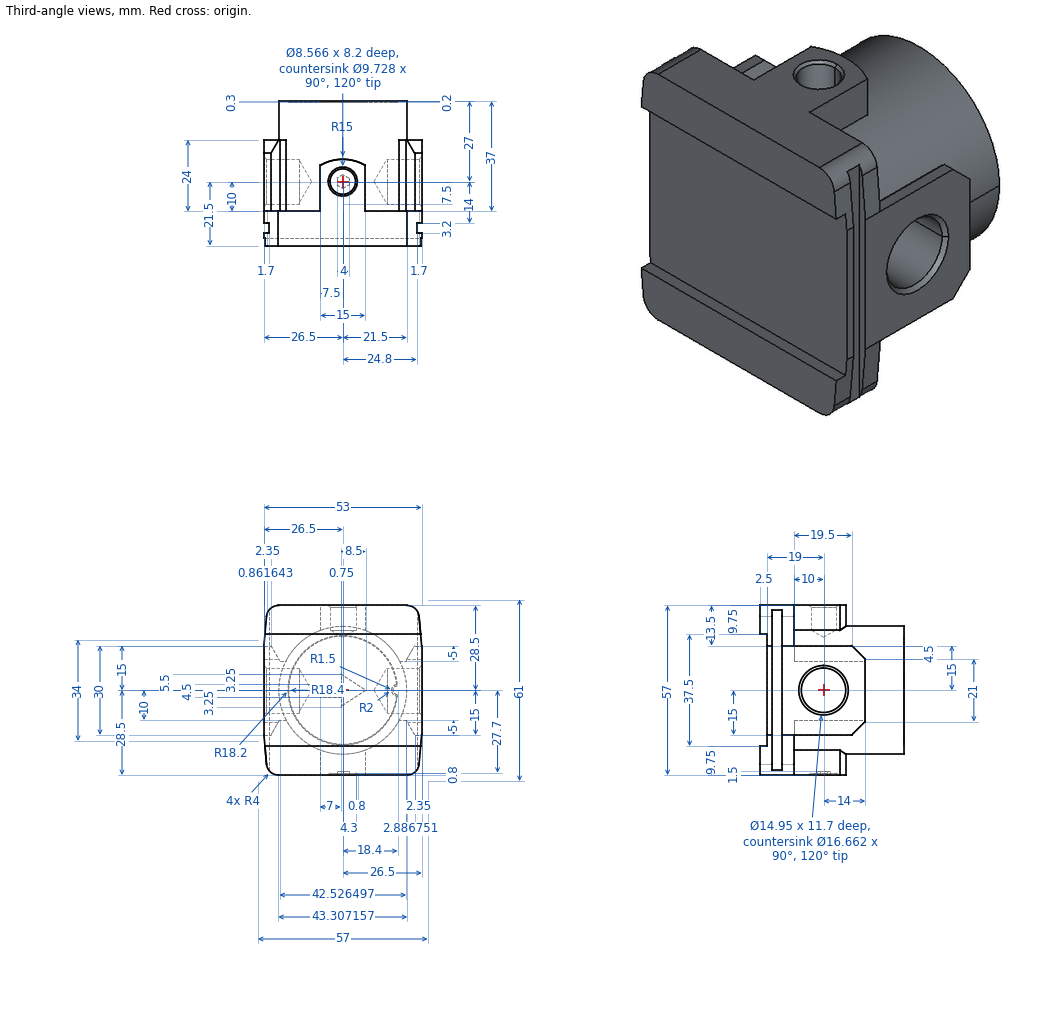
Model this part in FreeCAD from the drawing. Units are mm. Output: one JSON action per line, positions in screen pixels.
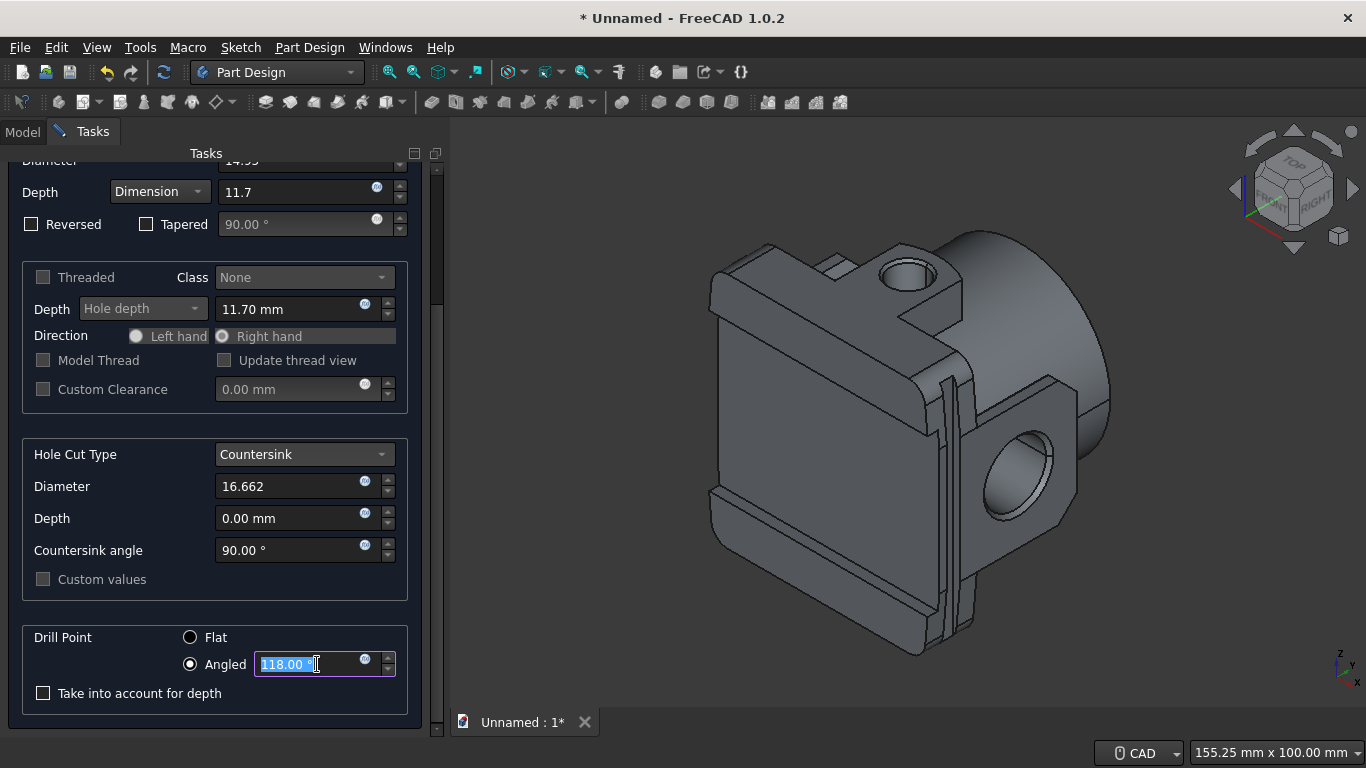
{"action": "type", "text": "120"}
{"action": "key", "text": "Tab"}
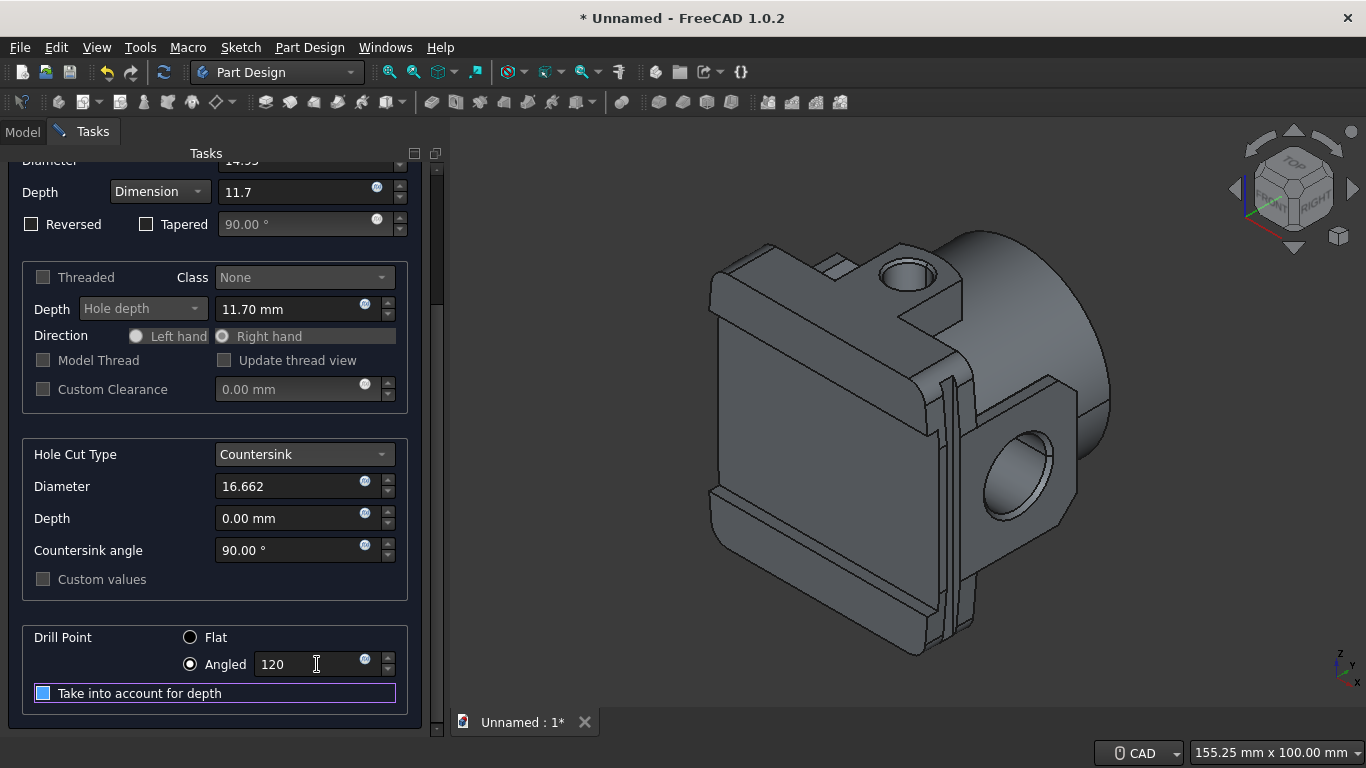
{"action": "scroll", "coordinate": [437, 450], "scroll_direction": "up", "scroll_amount": 4}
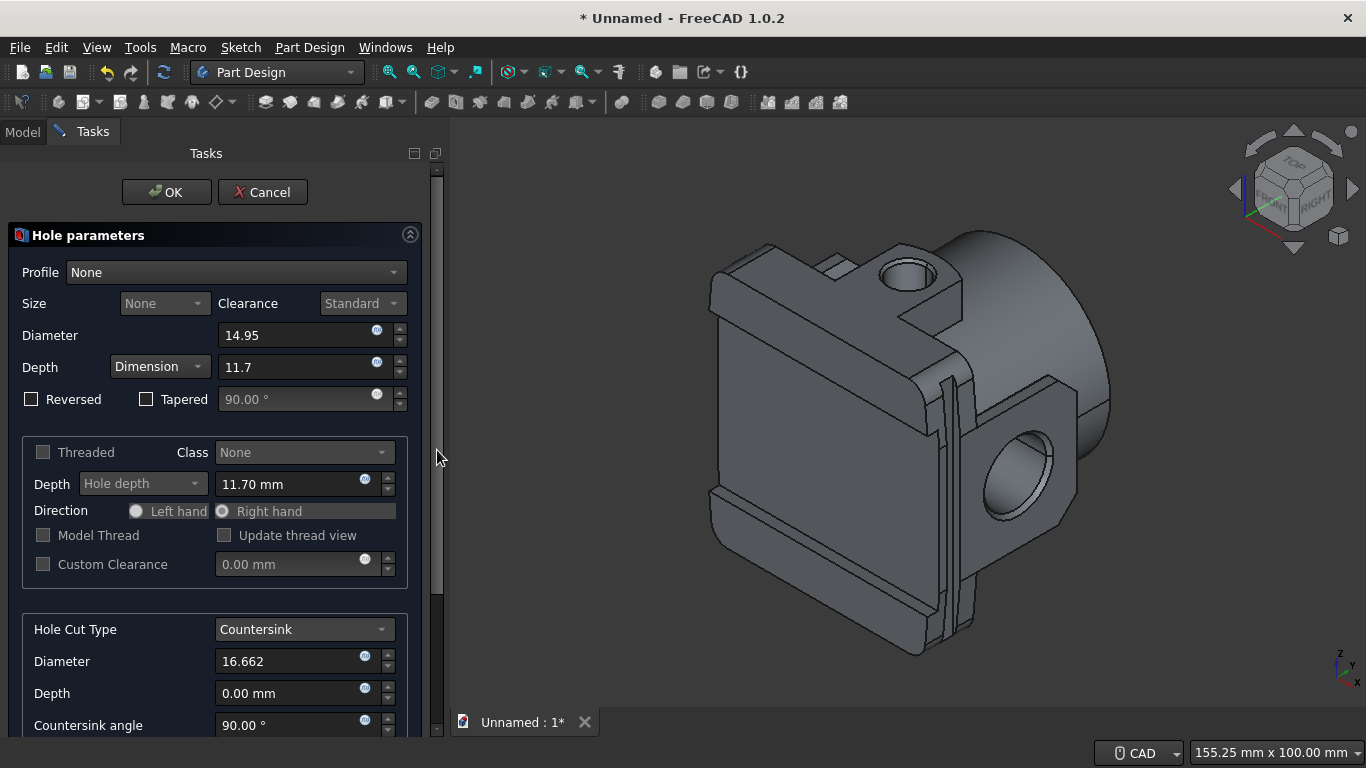
{"action": "left_click", "coordinate": [167, 192]}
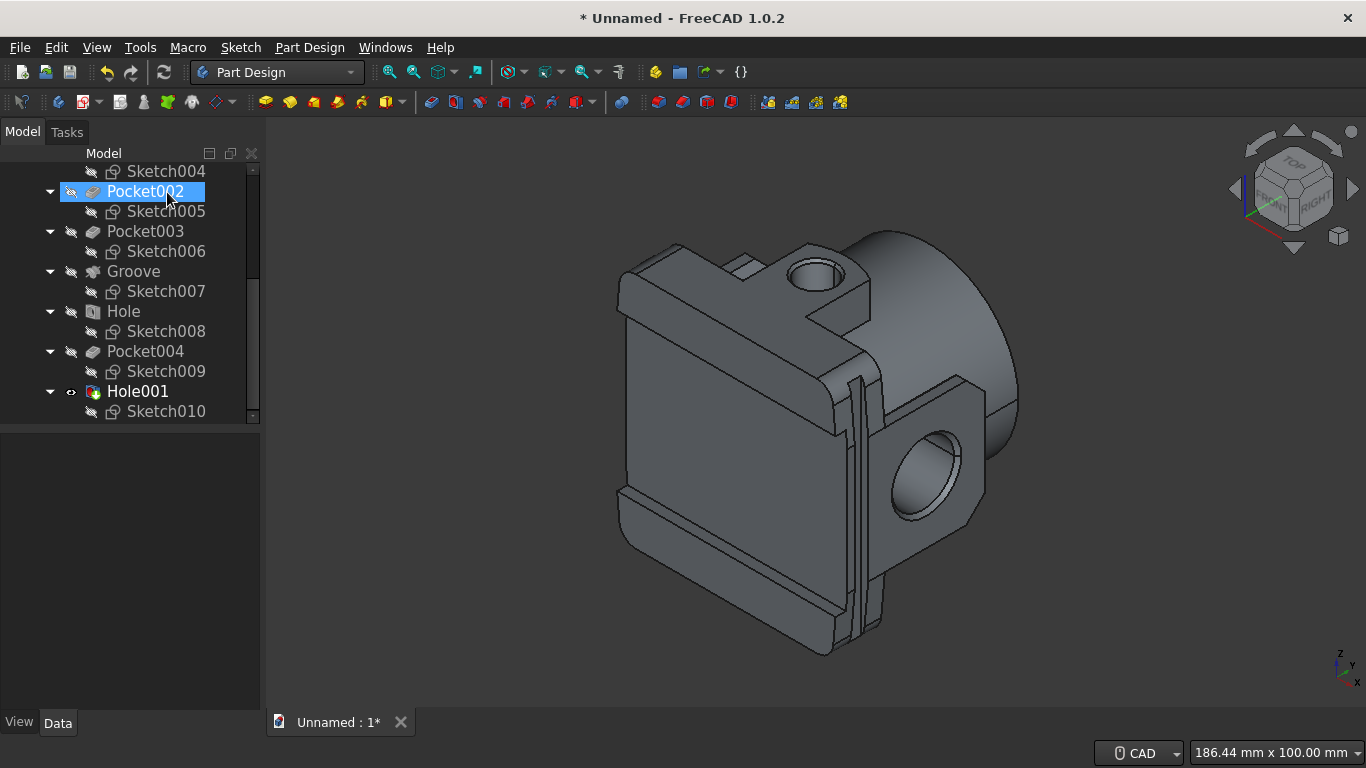
{"action": "key", "text": "6"}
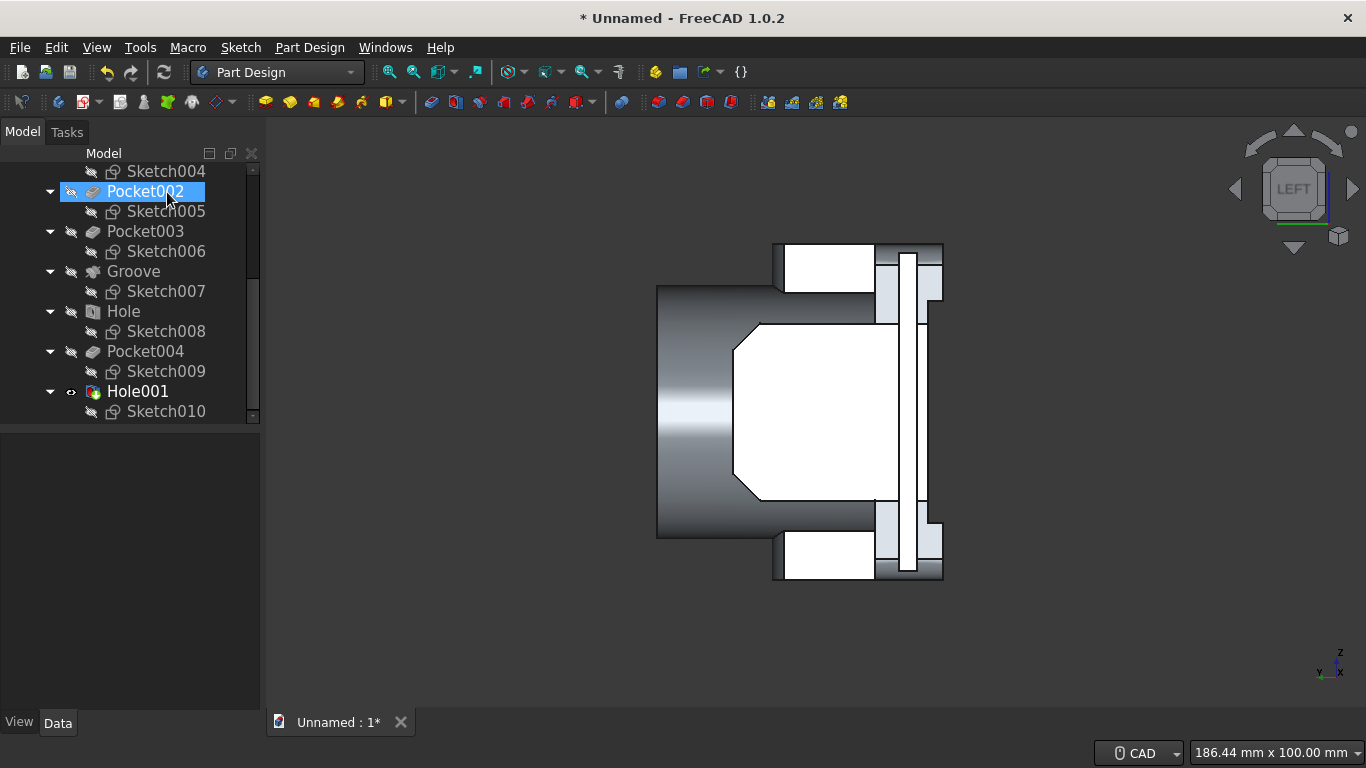
{"action": "left_click", "coordinate": [816, 411]}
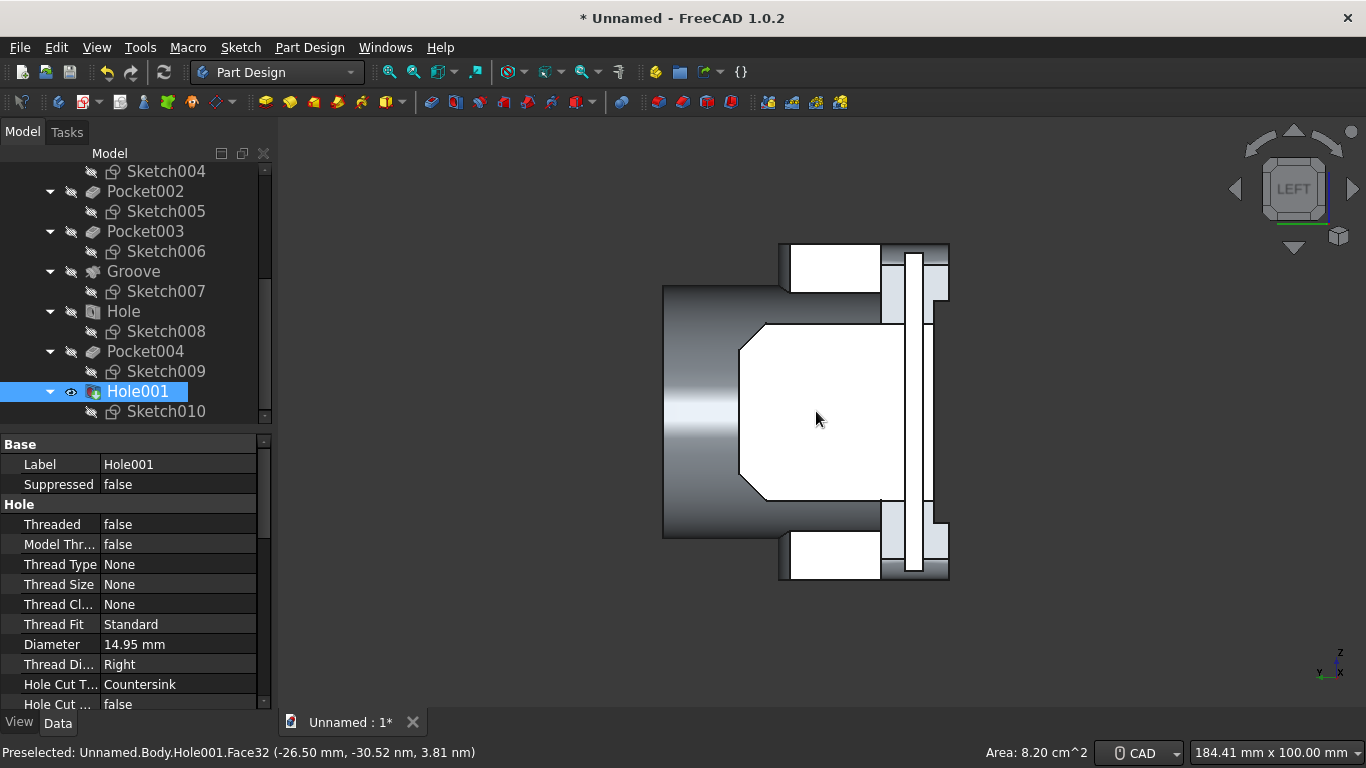
{"action": "left_click", "coordinate": [84, 102]}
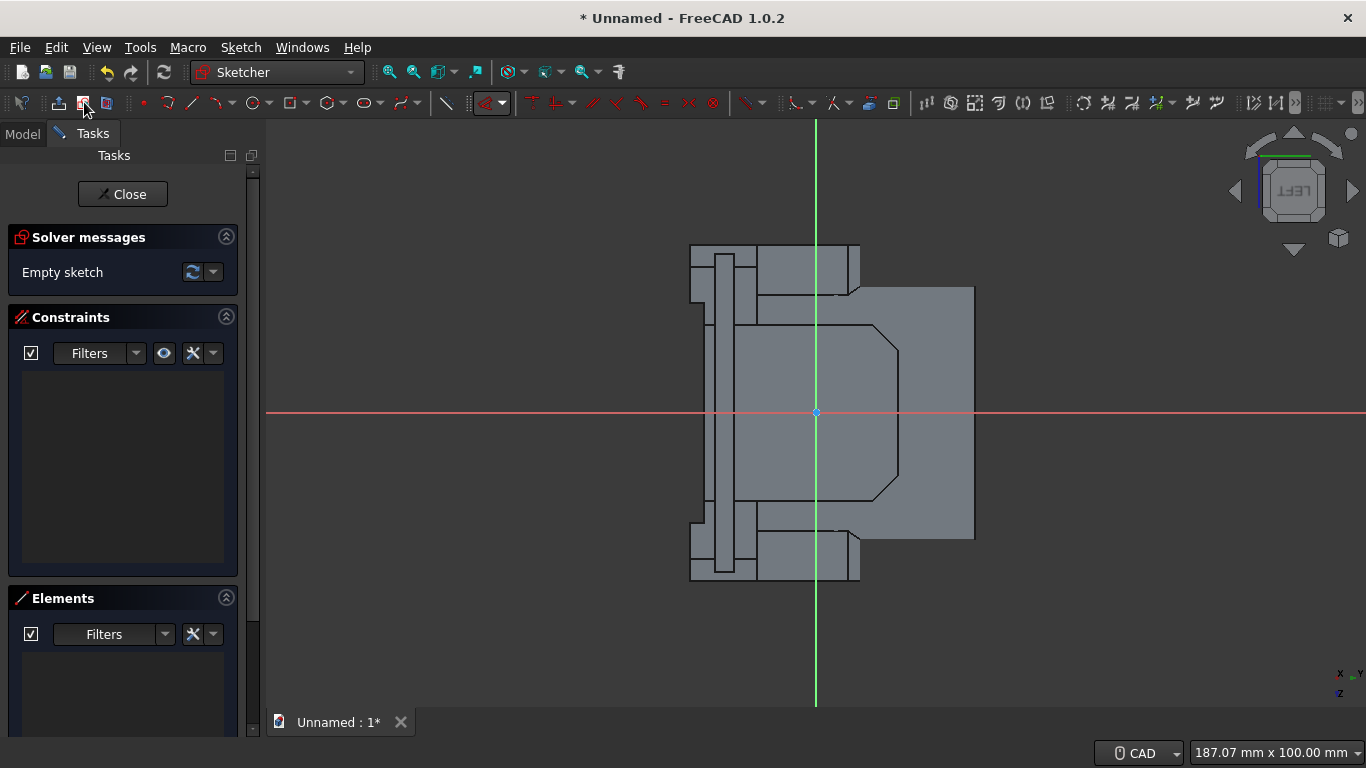
{"action": "scroll", "coordinate": [838, 413], "scroll_direction": "up", "scroll_amount": 7}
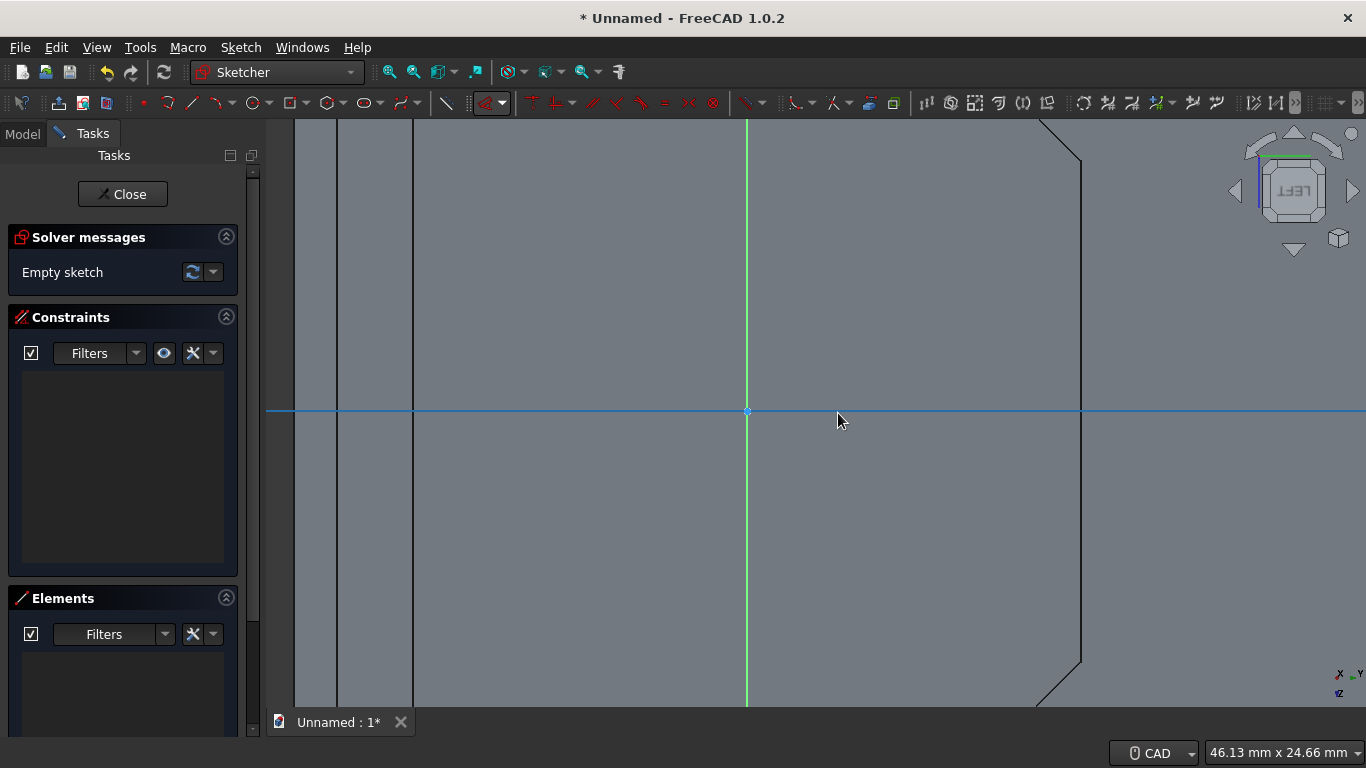
{"action": "left_click", "coordinate": [254, 104]}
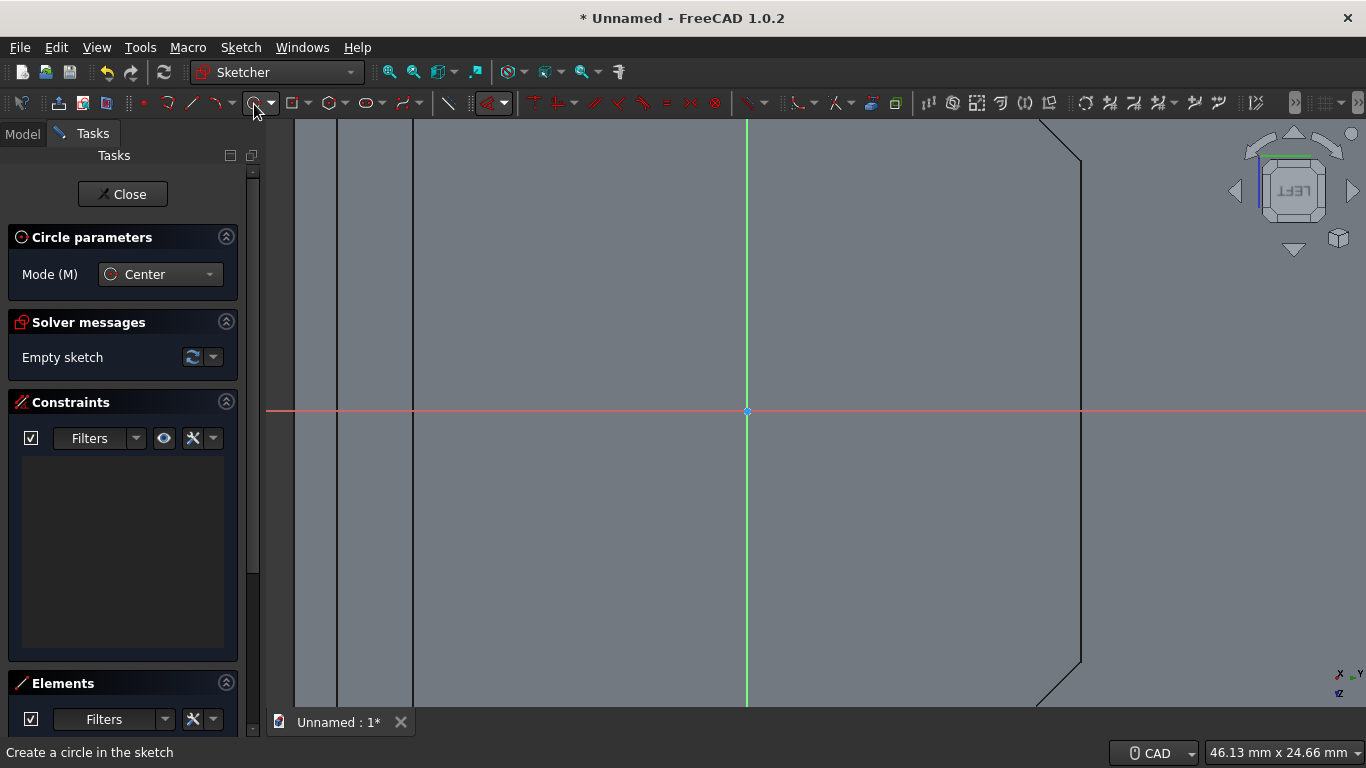
{"action": "left_click", "coordinate": [747, 411]}
{"action": "mouse_move", "coordinate": [873, 285]}